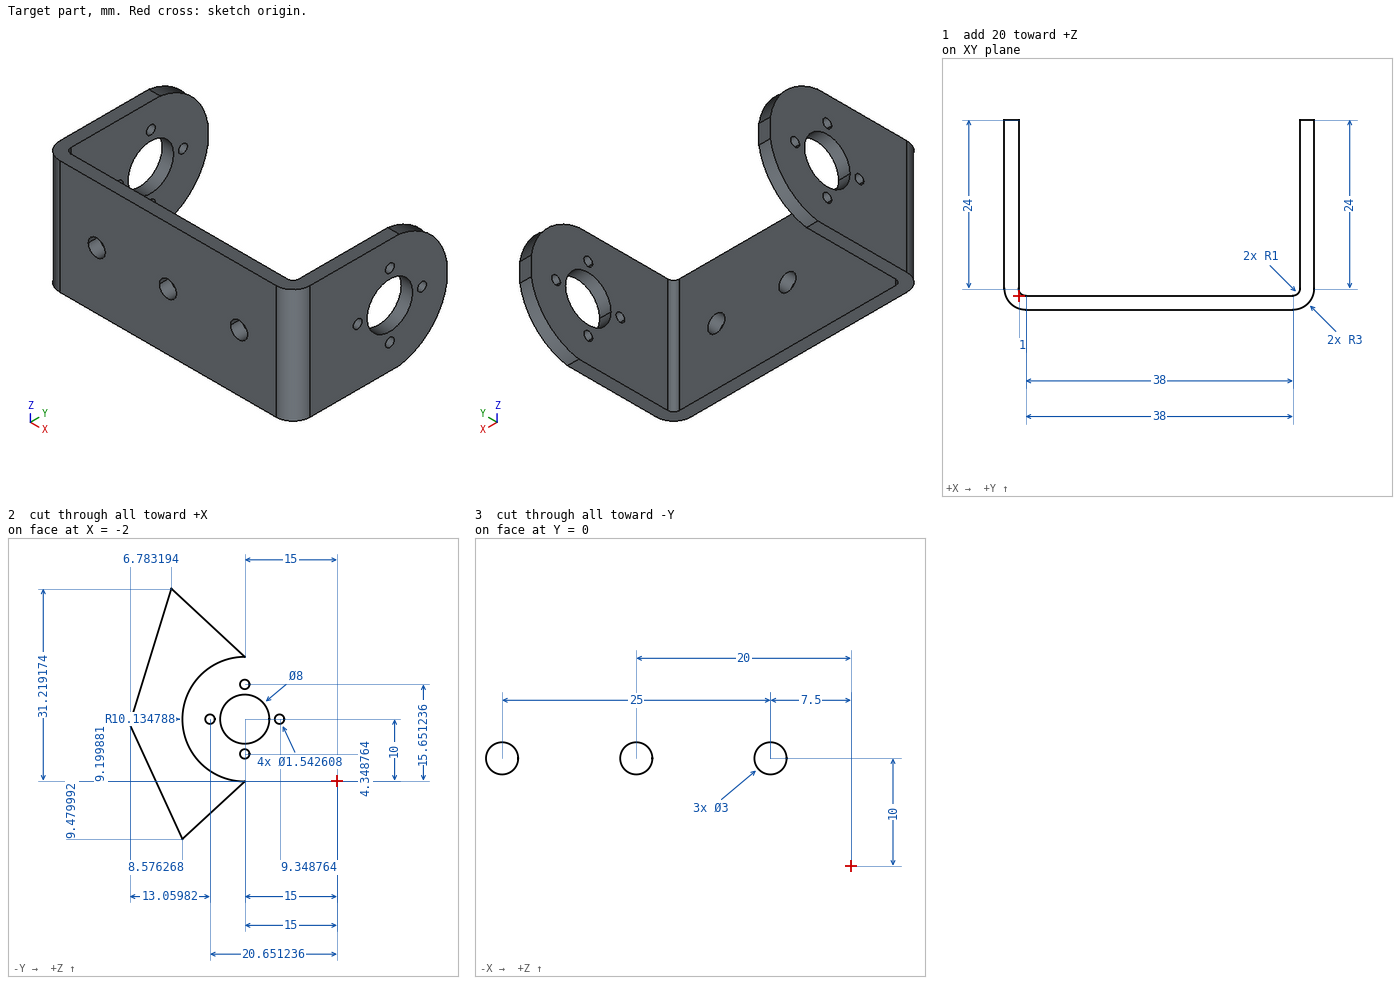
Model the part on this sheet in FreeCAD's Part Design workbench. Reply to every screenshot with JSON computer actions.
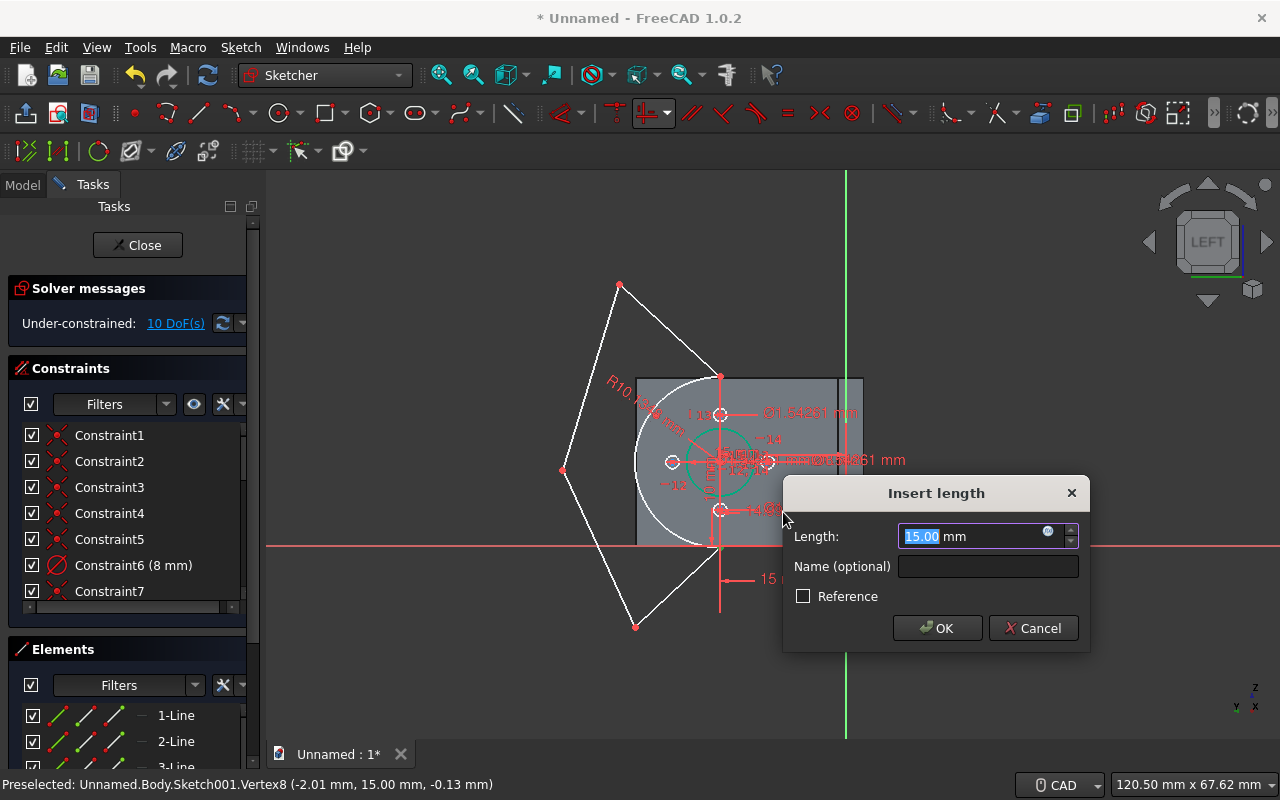
{"action": "type", "text": "15"}
{"action": "key", "text": "Return"}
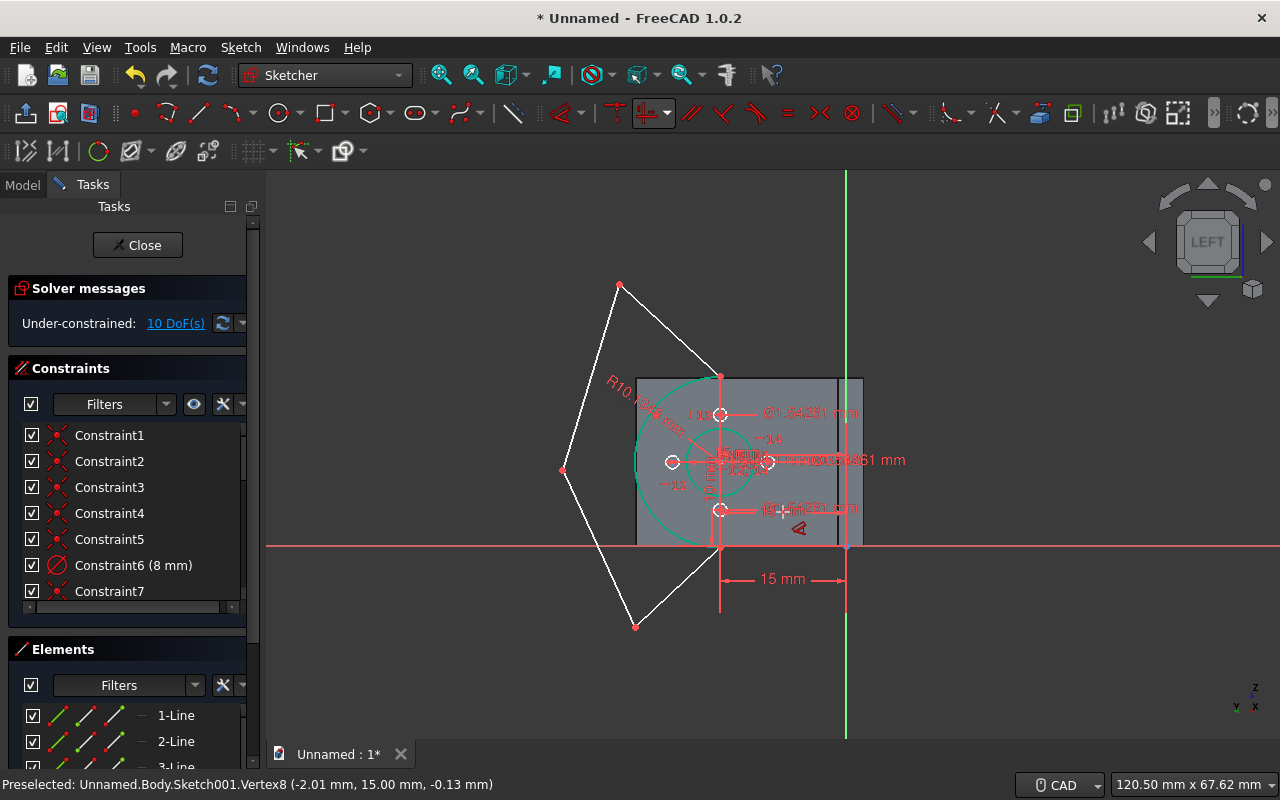
{"action": "left_click", "coordinate": [768, 462]}
{"action": "left_click", "coordinate": [807, 428]}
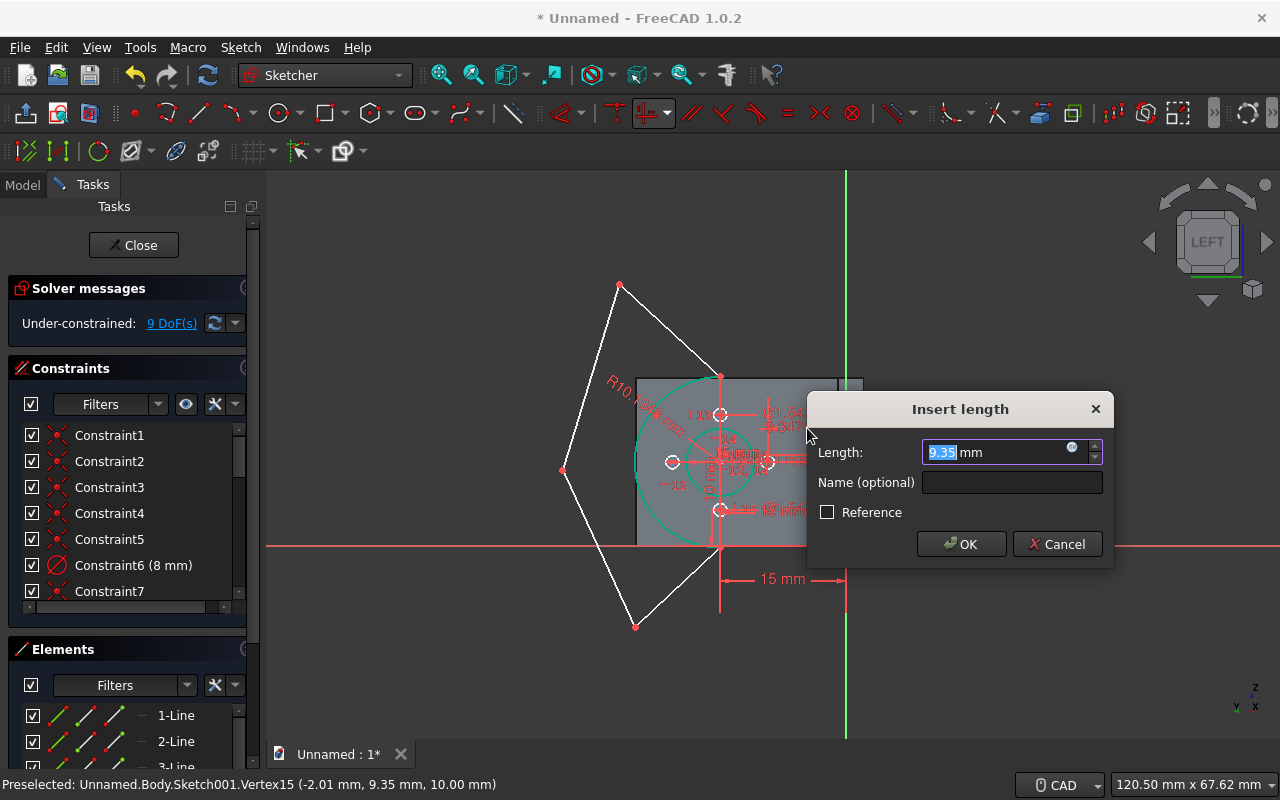
{"action": "type", "text": "9.348764"}
{"action": "key", "text": "Return"}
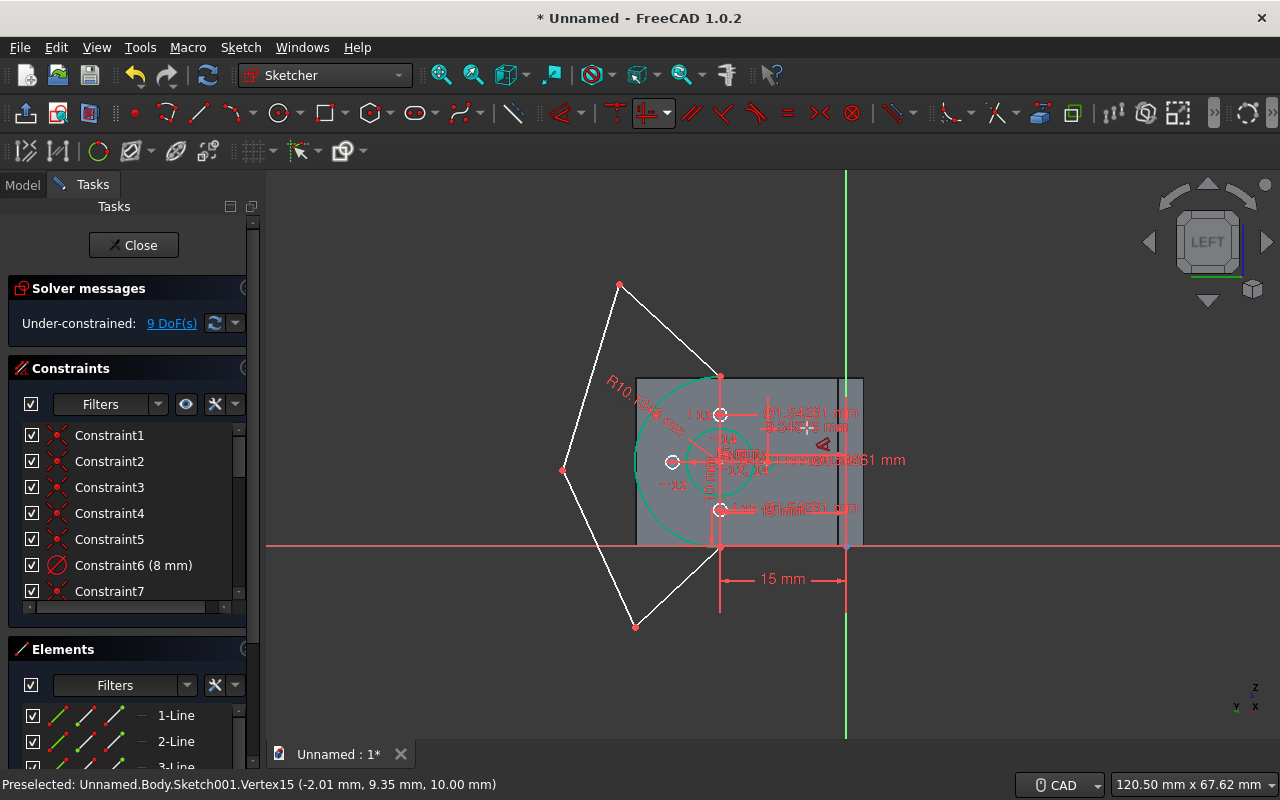
{"action": "left_click", "coordinate": [720, 510]}
{"action": "left_click", "coordinate": [880, 528]}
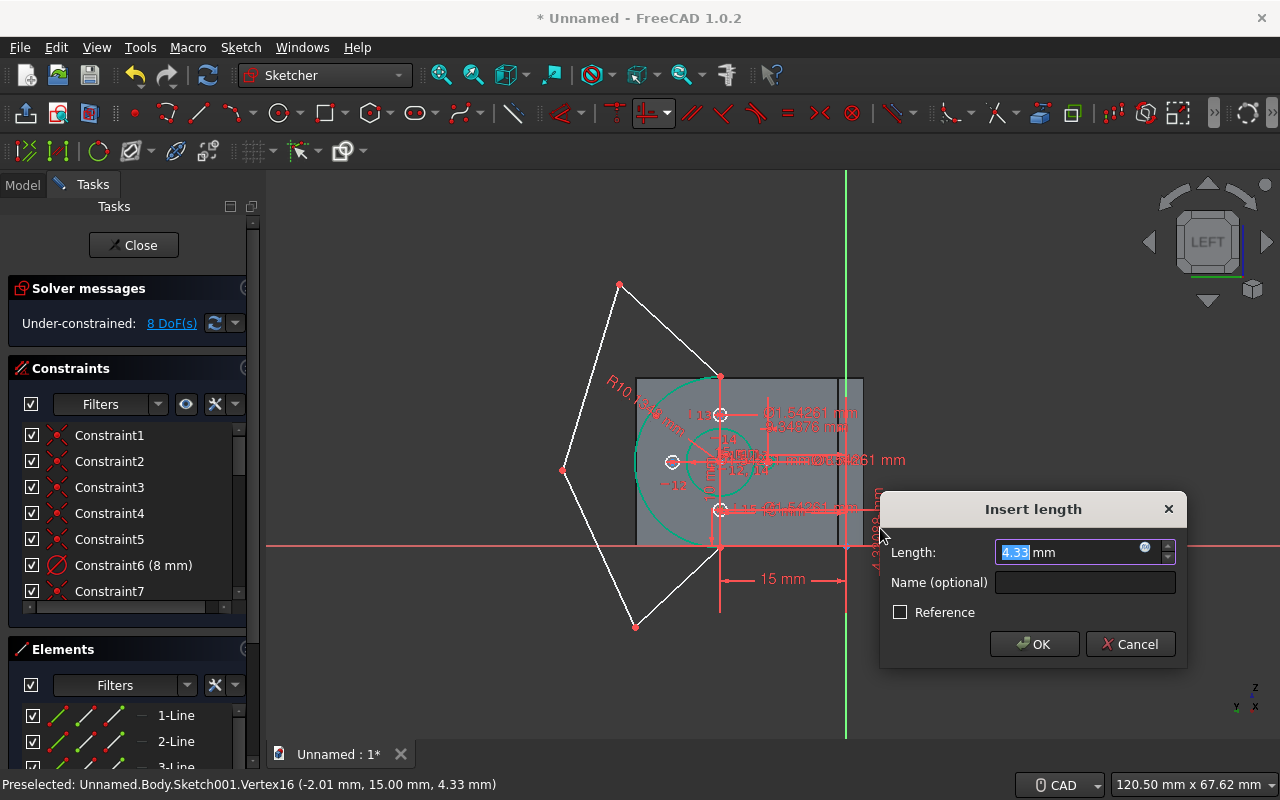
{"action": "type", "text": "4.348764"}
{"action": "key", "text": "Return"}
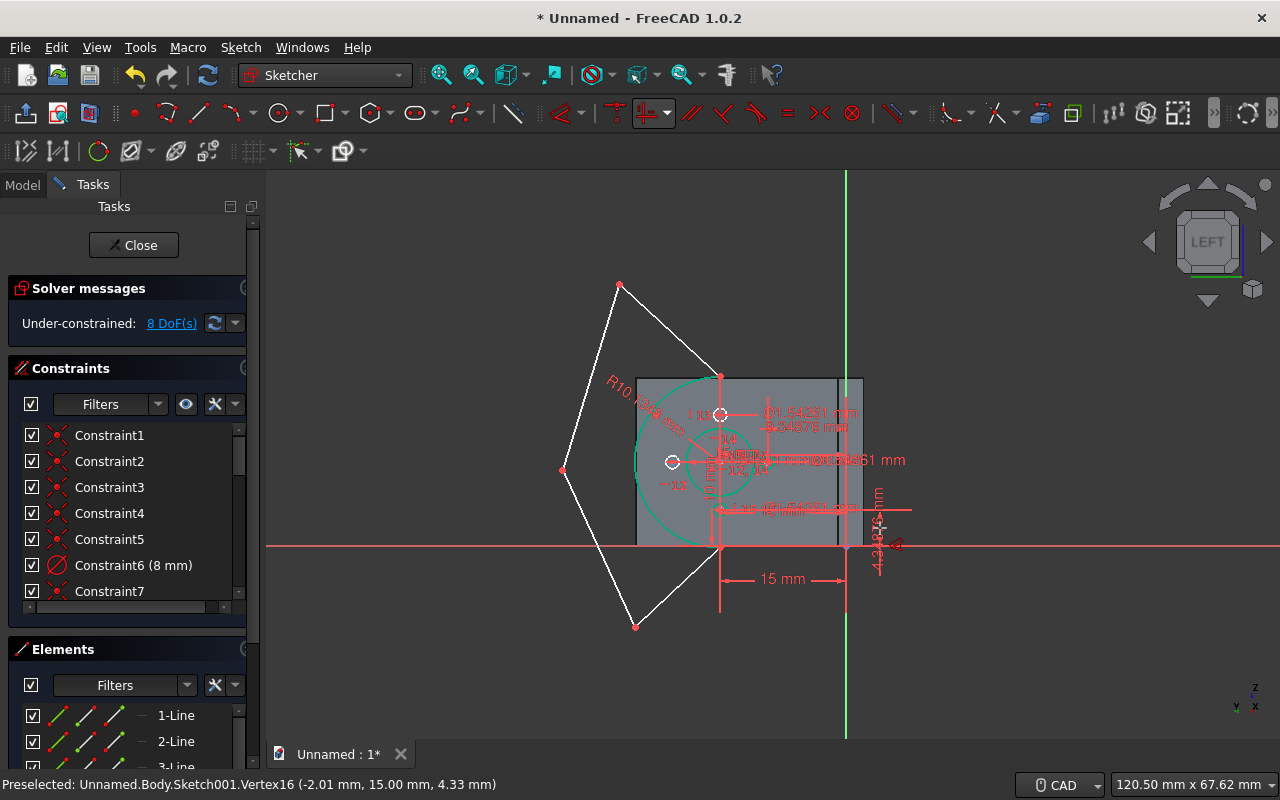
{"action": "left_click", "coordinate": [563, 470]}
{"action": "left_click", "coordinate": [880, 491]}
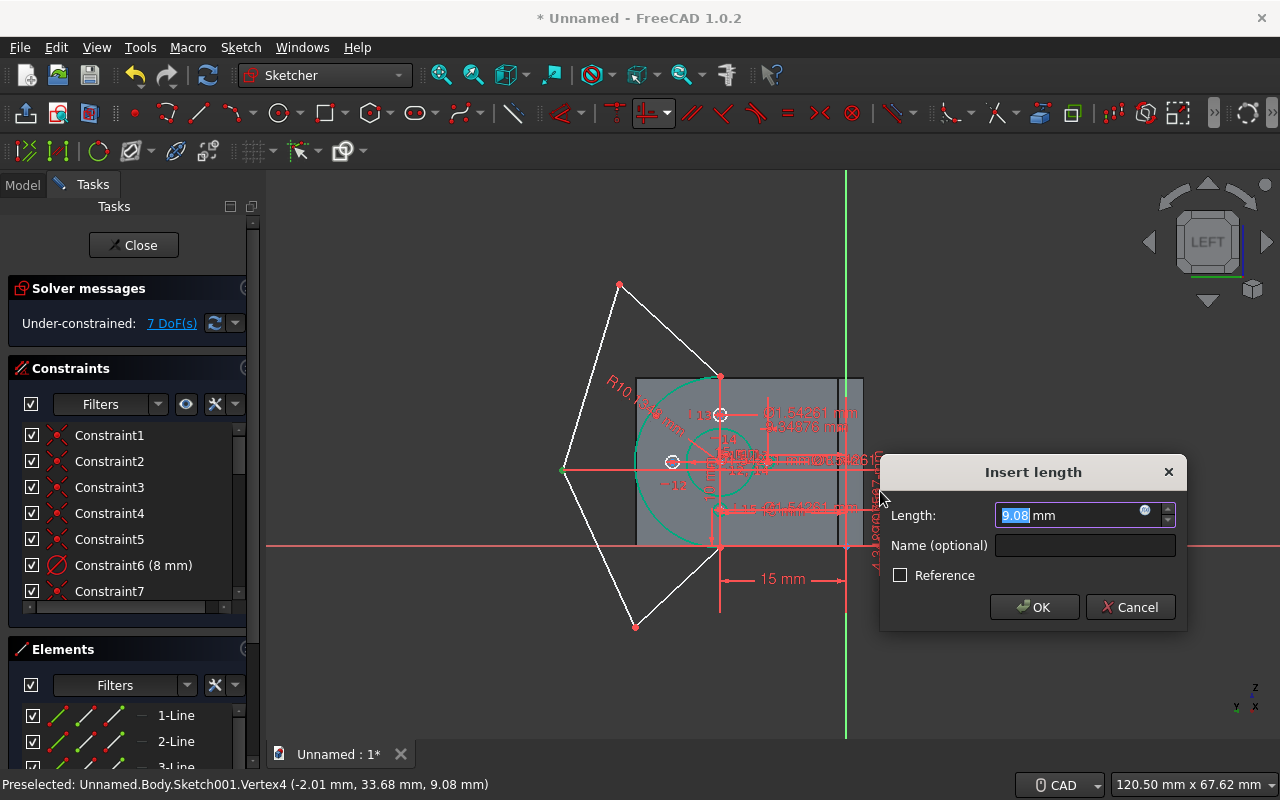
{"action": "type", "text": "9.199881"}
{"action": "key", "text": "Return"}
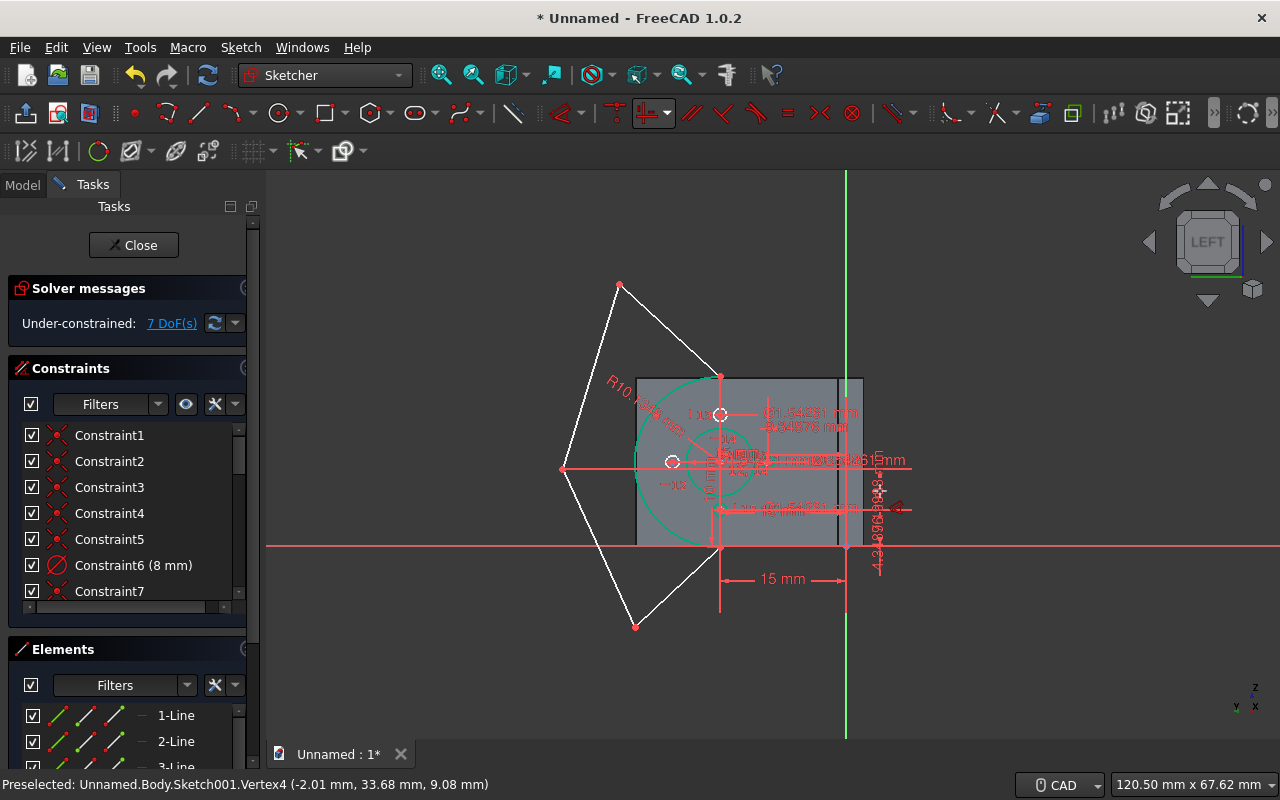
{"action": "left_click", "coordinate": [635, 627]}
{"action": "left_click", "coordinate": [880, 587]}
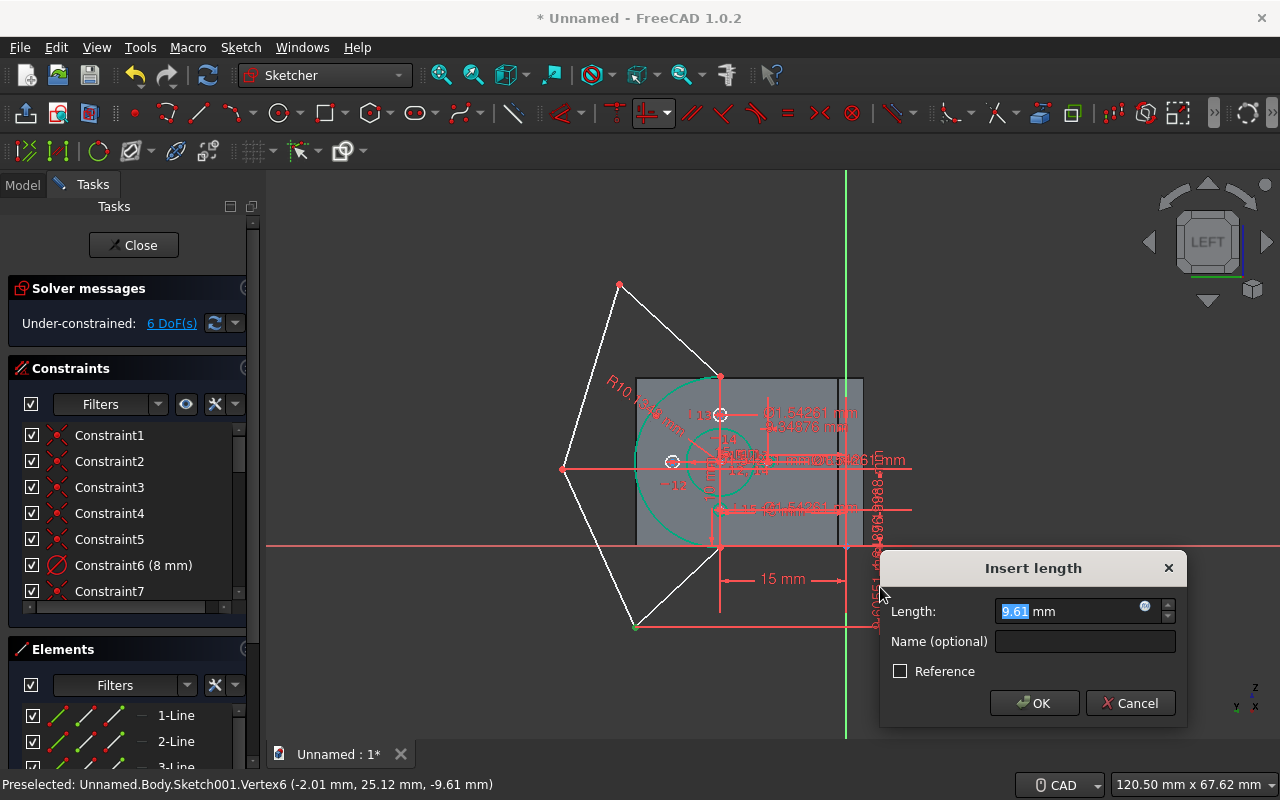
{"action": "type", "text": "9.479992"}
{"action": "key", "text": "Return"}